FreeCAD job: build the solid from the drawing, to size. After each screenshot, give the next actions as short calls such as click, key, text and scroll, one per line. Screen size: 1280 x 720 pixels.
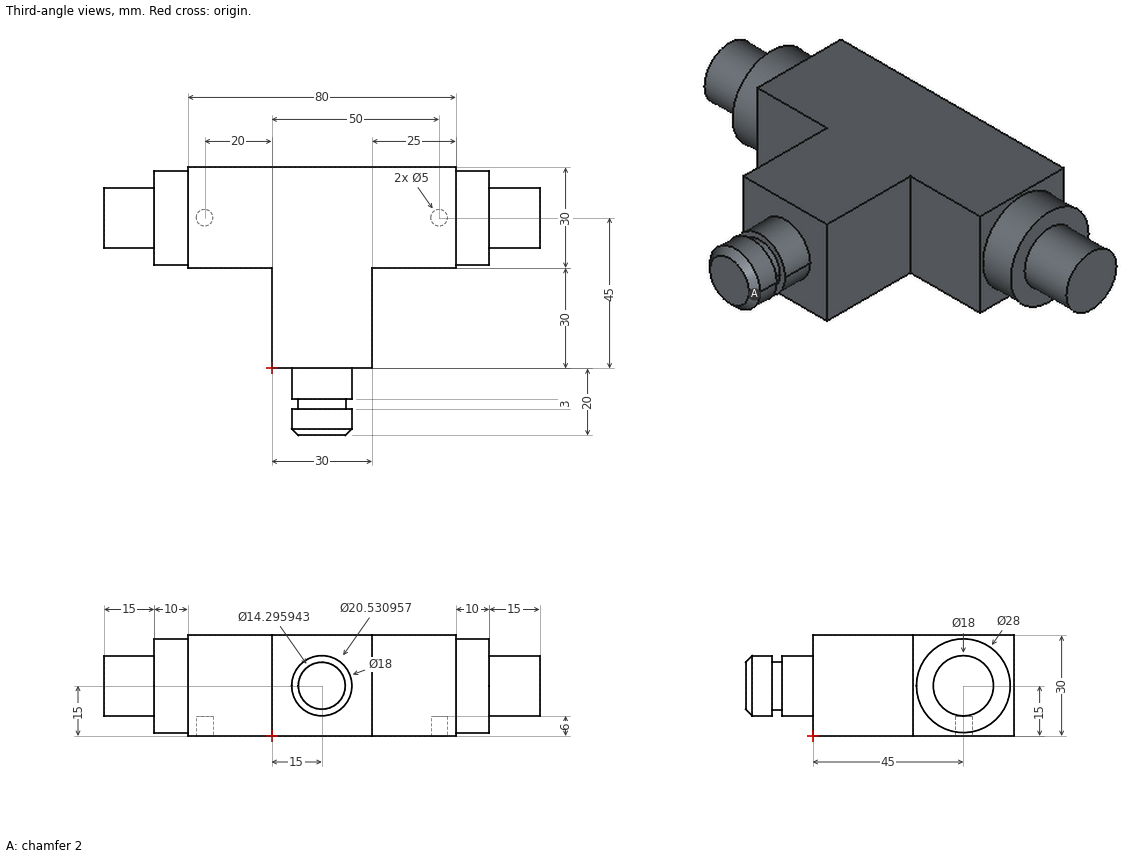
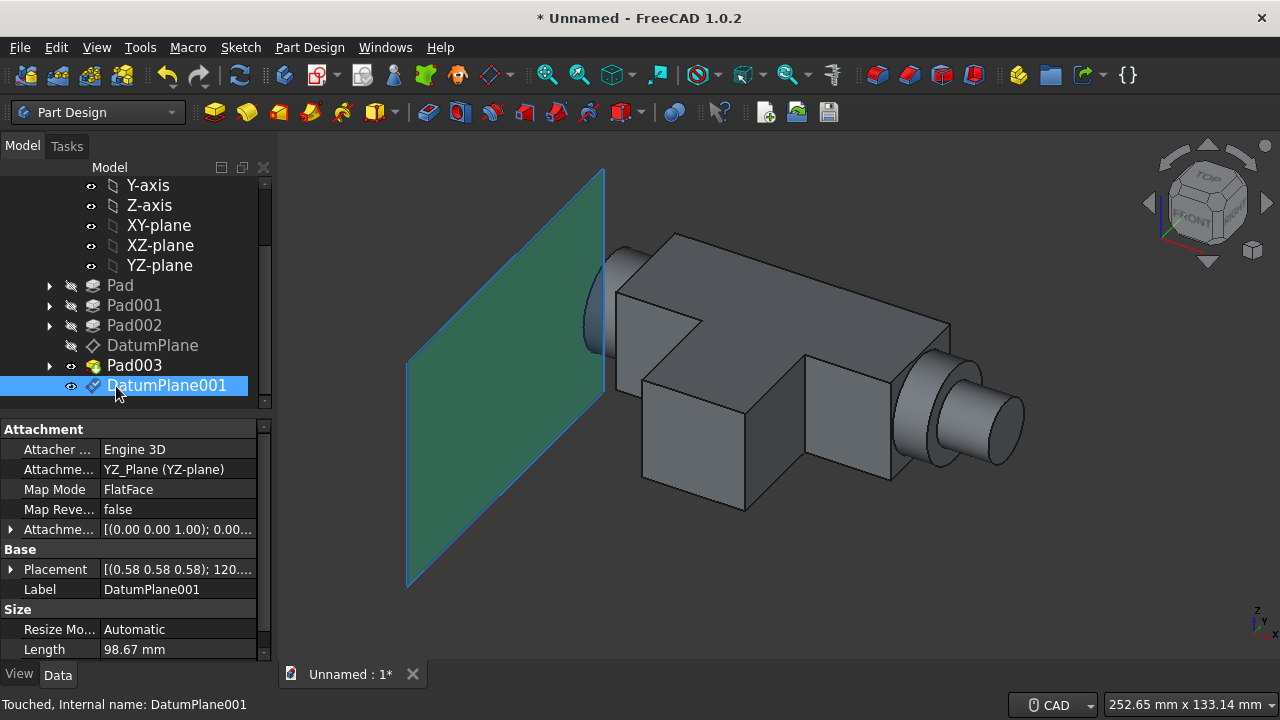
click(318, 76)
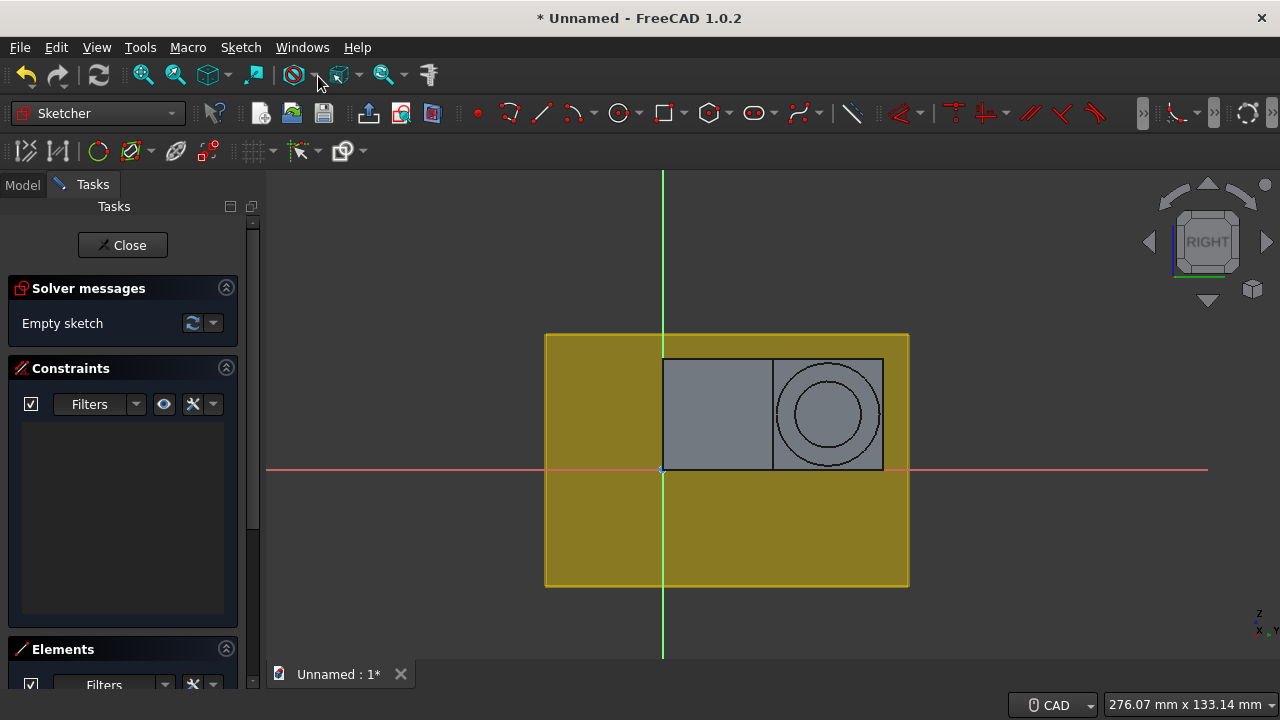
key(q)
key(s)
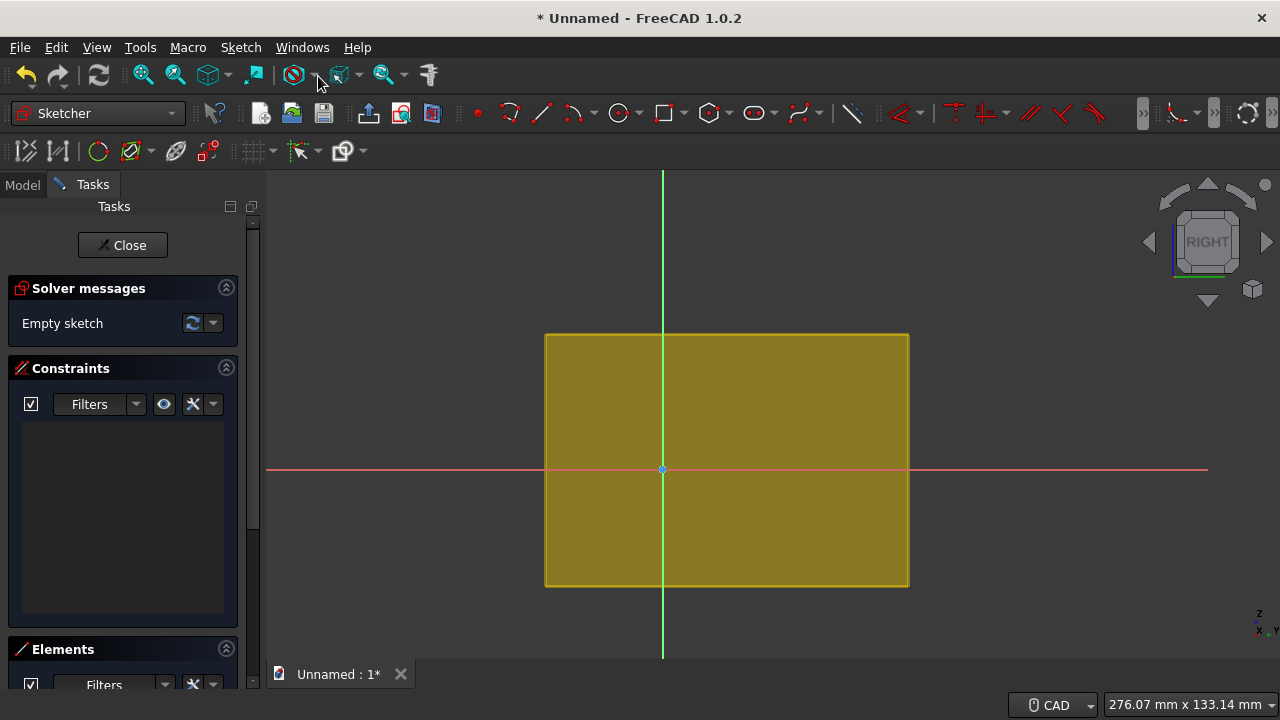
scroll(859, 414, up, 8)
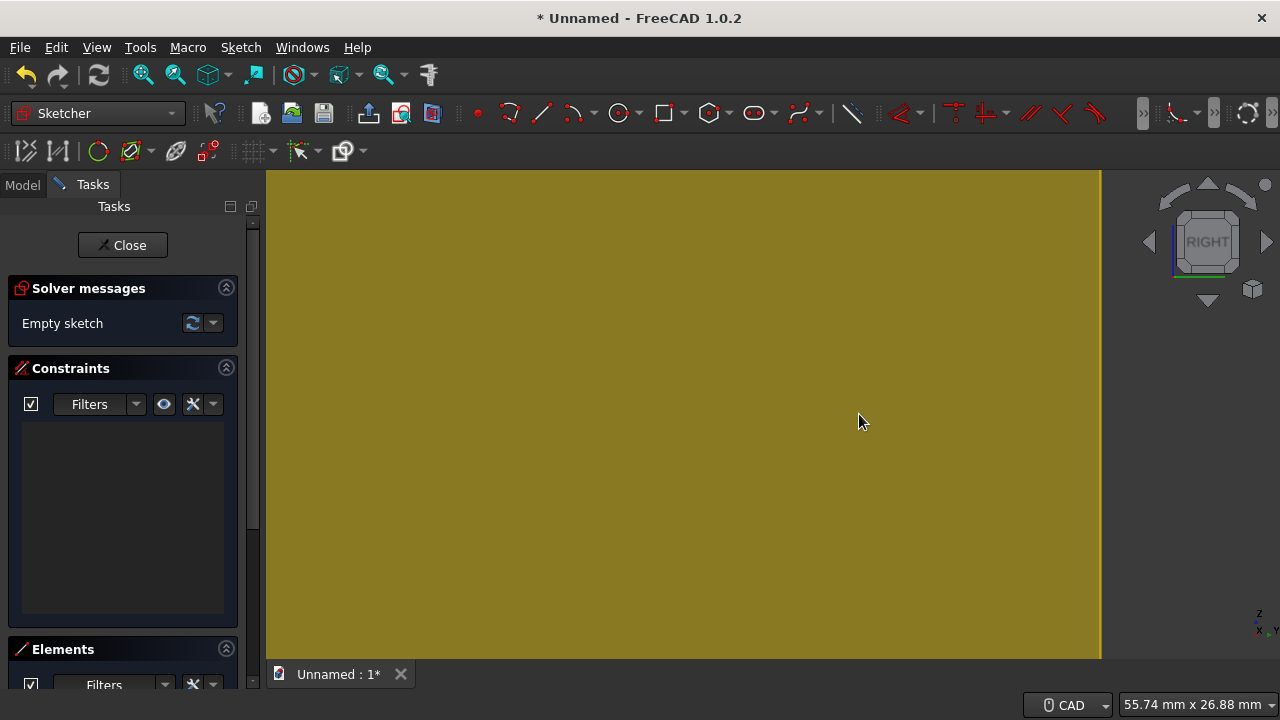
key(g)
key(c)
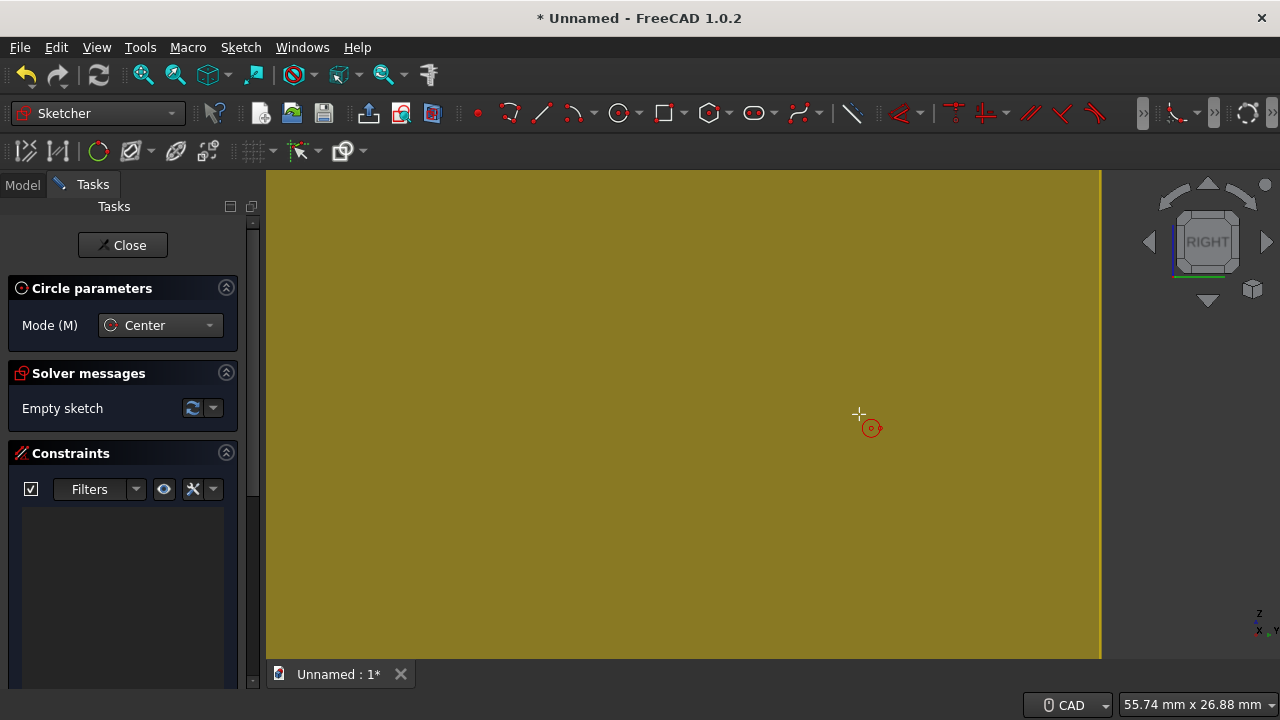
click(704, 415)
move(819, 299)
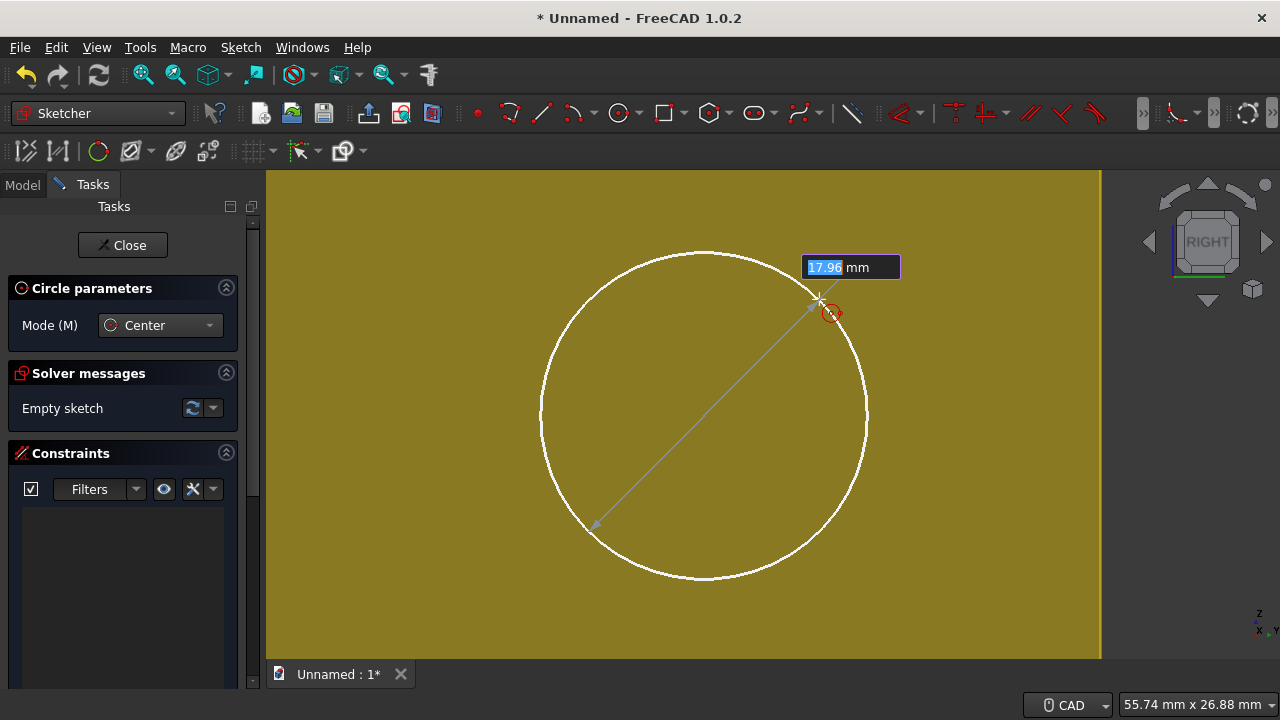
text(18)
key(Return)
key(Escape)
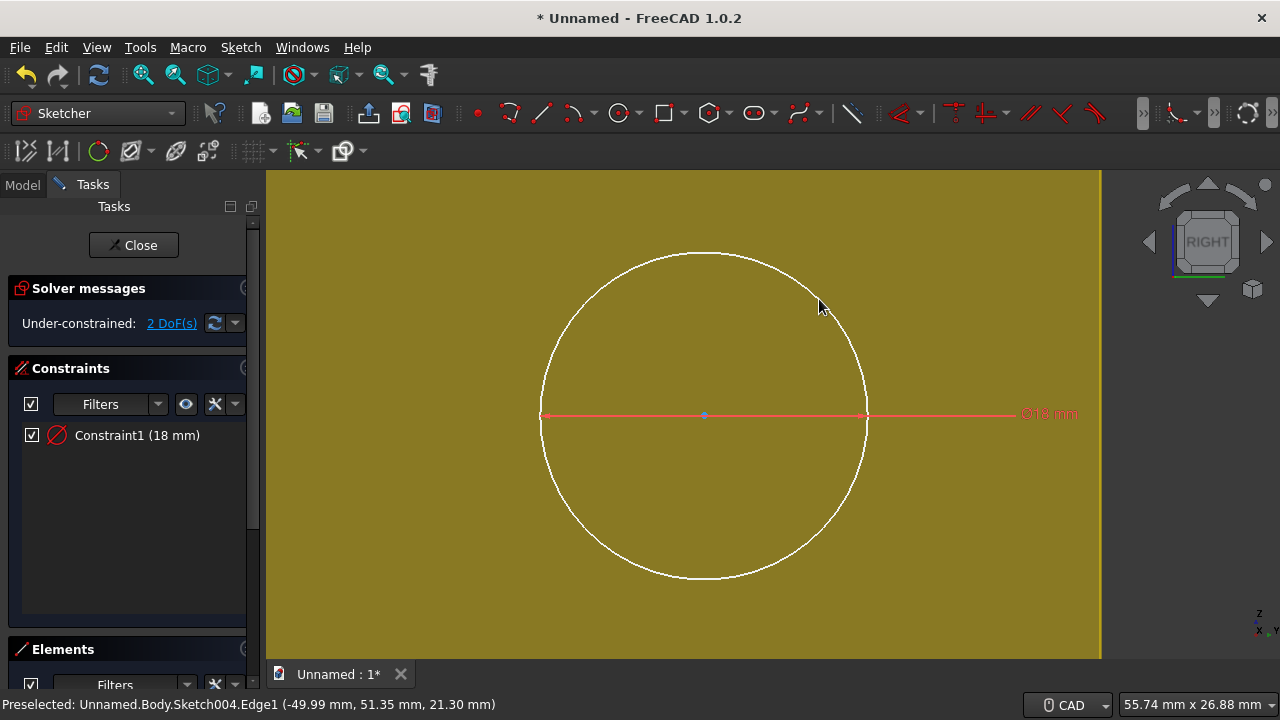
key(d)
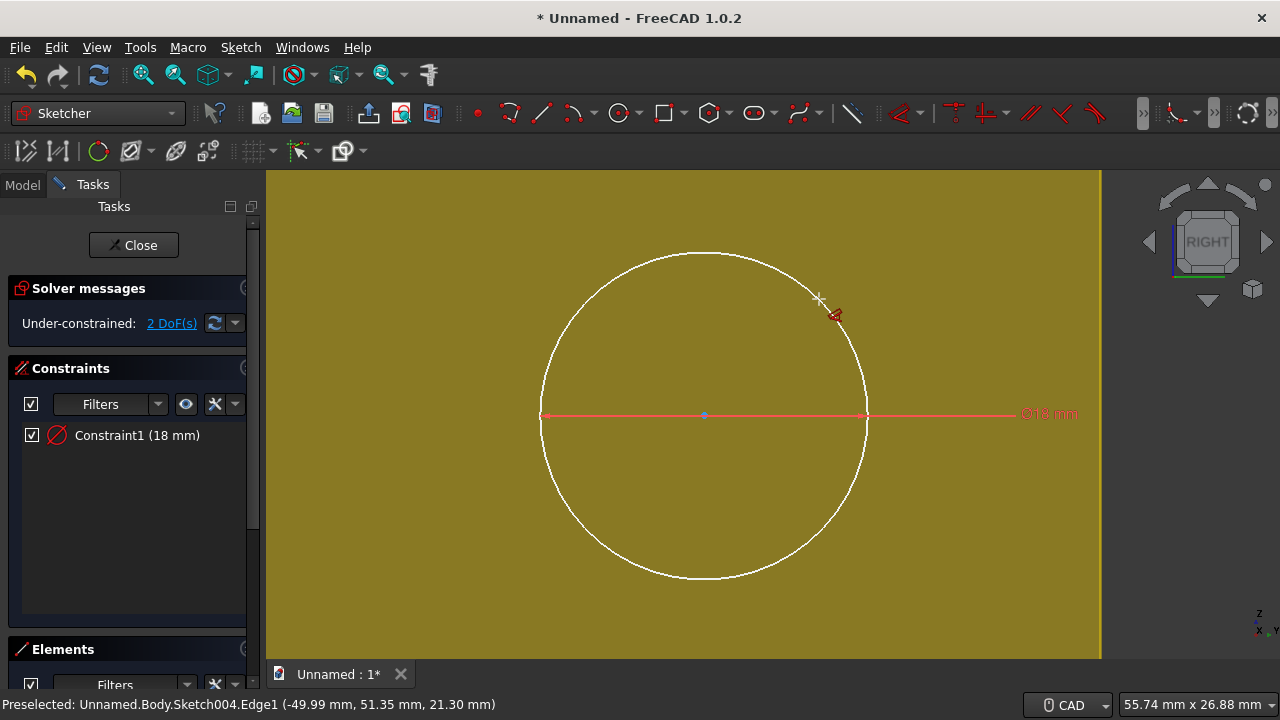
click(704, 416)
click(499, 382)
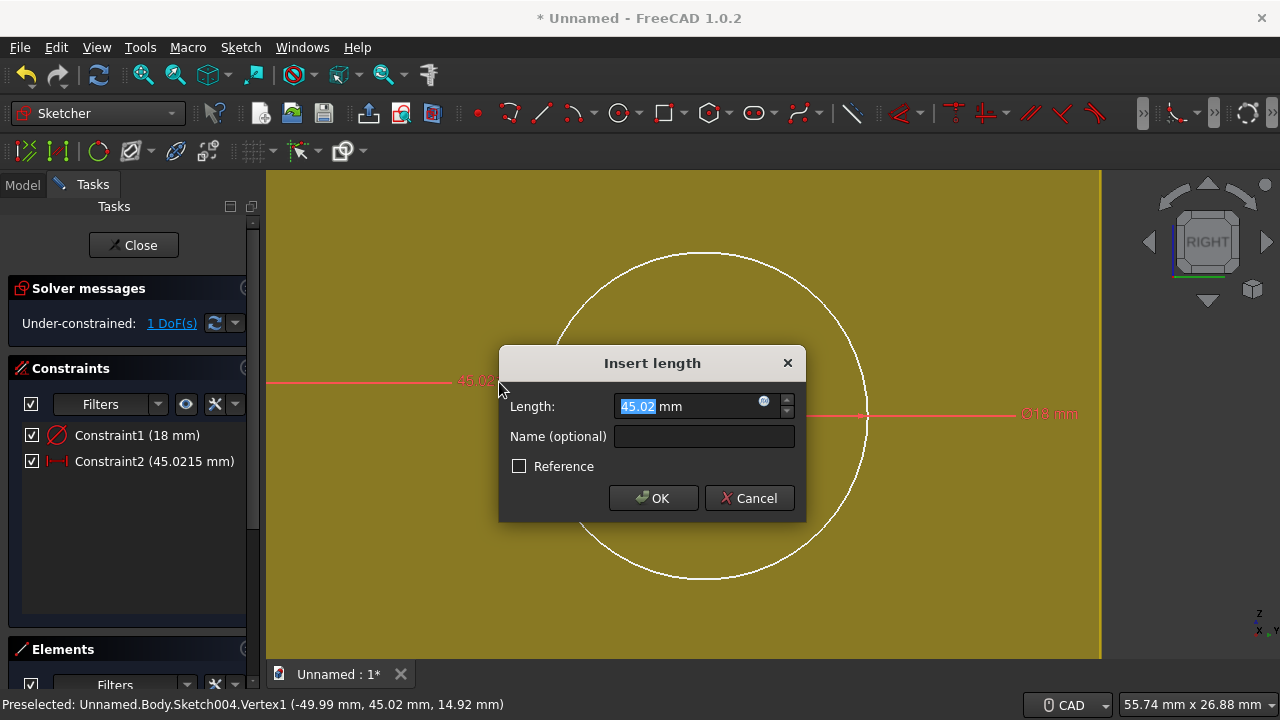
text(45)
key(Return)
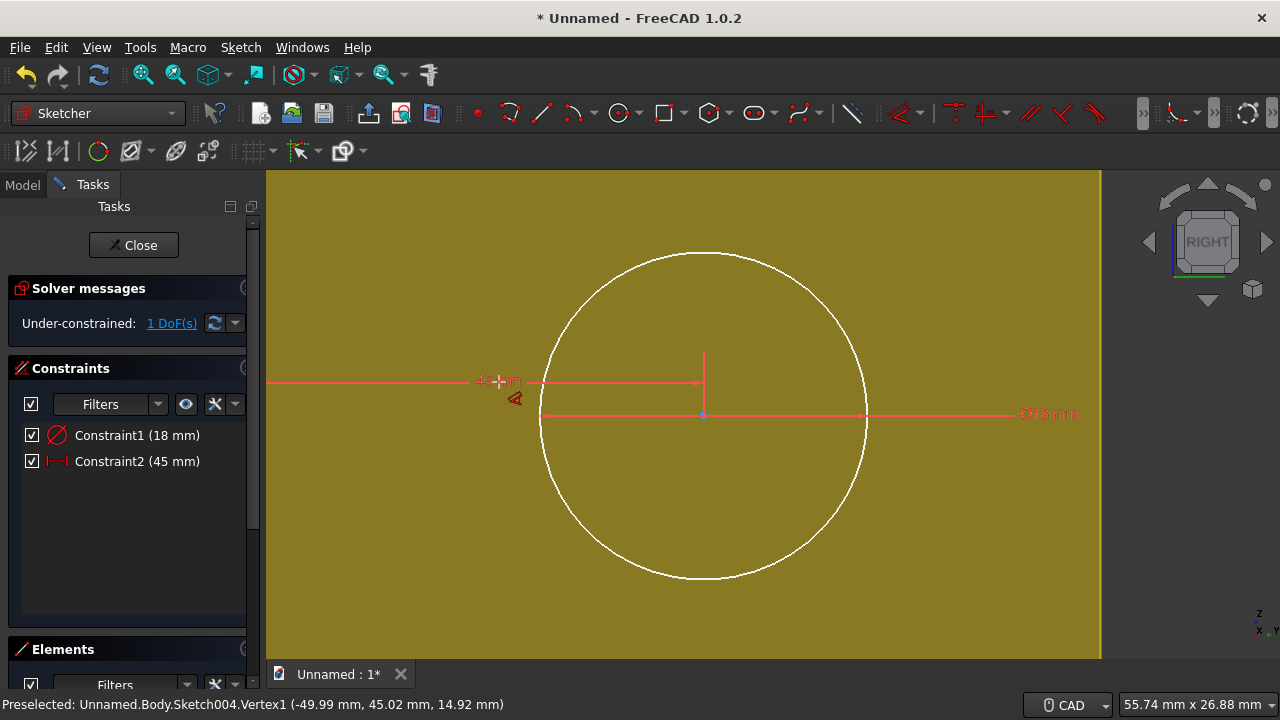
click(704, 416)
click(738, 524)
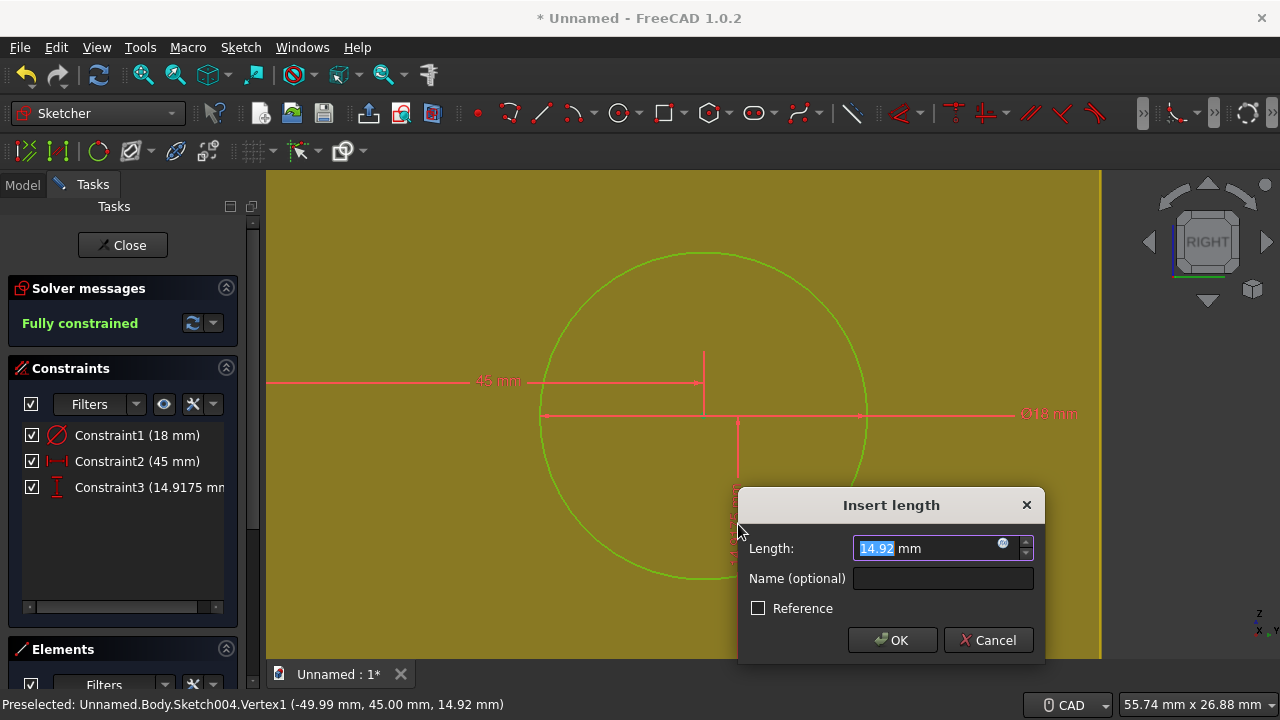
text(15)
key(Return)
key(Escape)